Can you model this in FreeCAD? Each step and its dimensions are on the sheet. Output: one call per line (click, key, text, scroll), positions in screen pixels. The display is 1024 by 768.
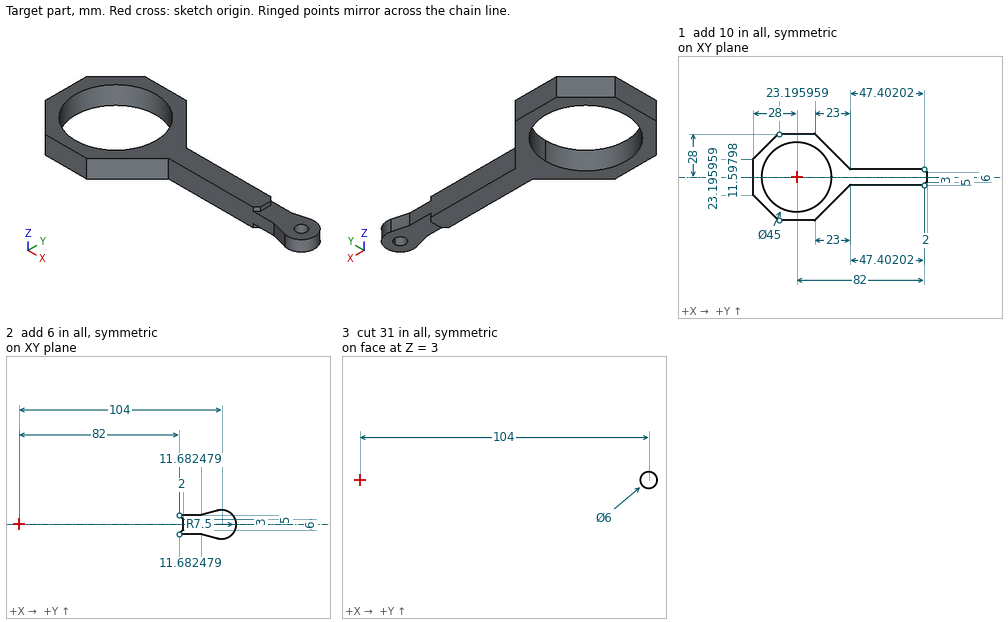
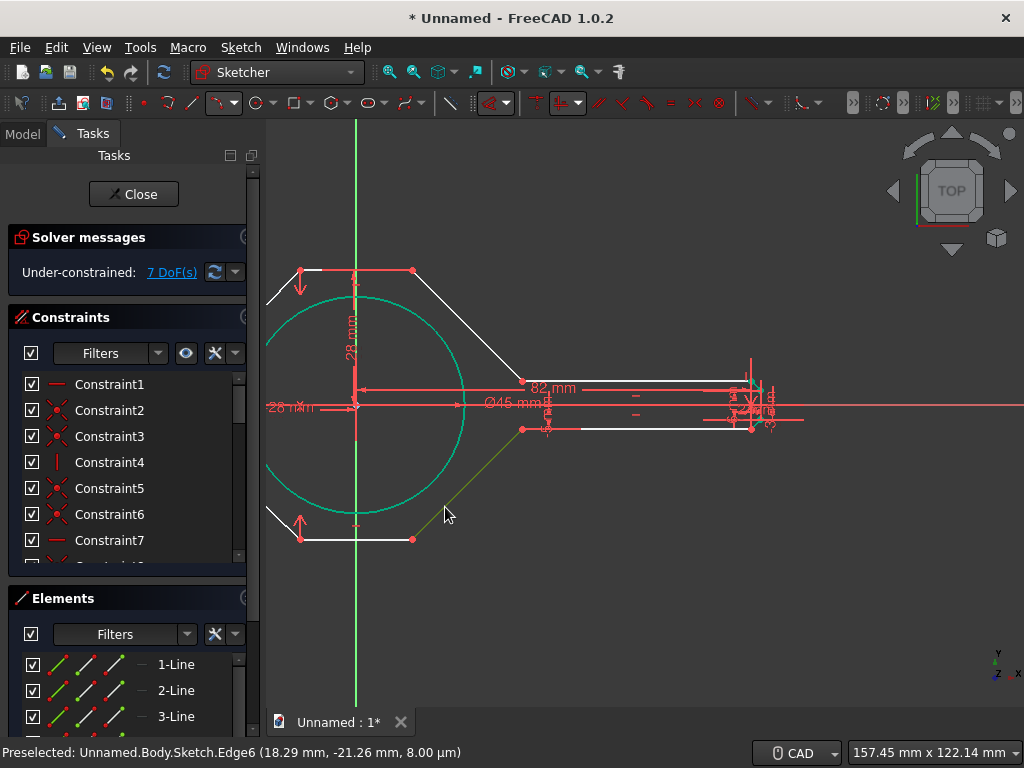
click(508, 104)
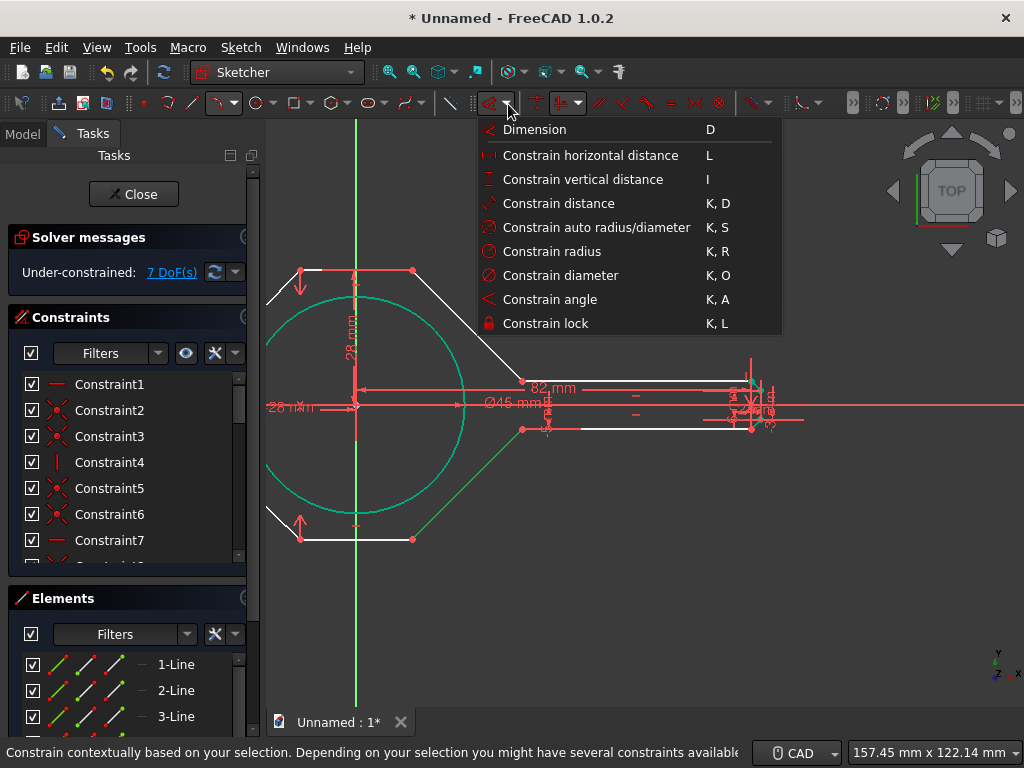
click(630, 155)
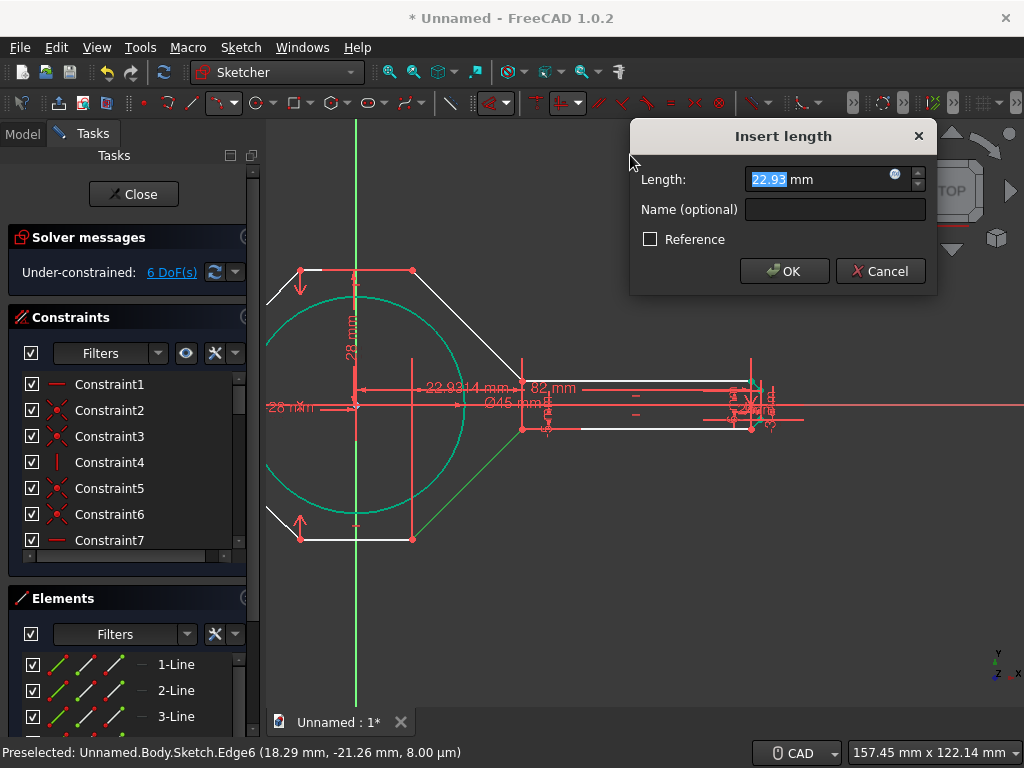
text(23)
key(Return)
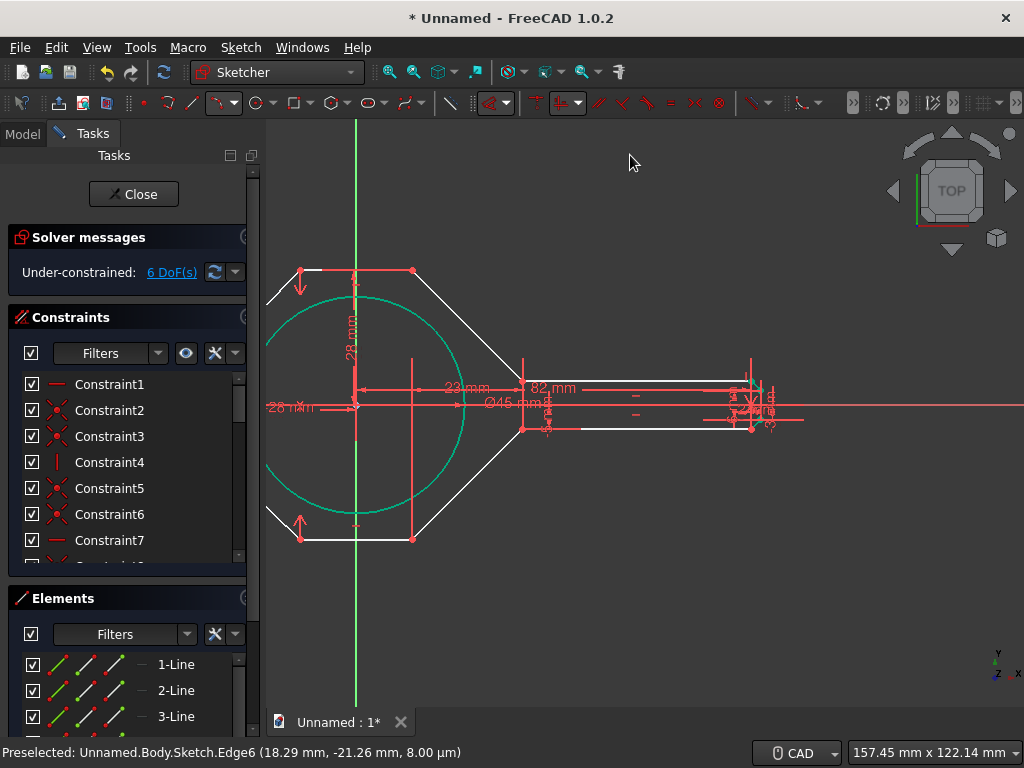
click(489, 348)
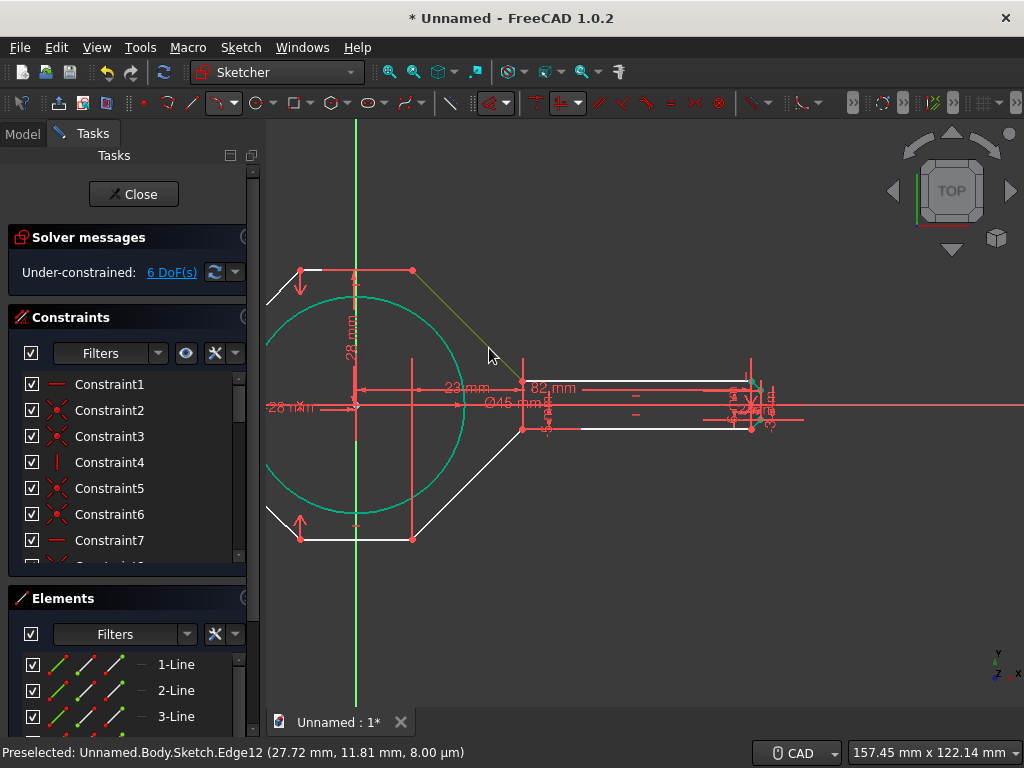
key(l)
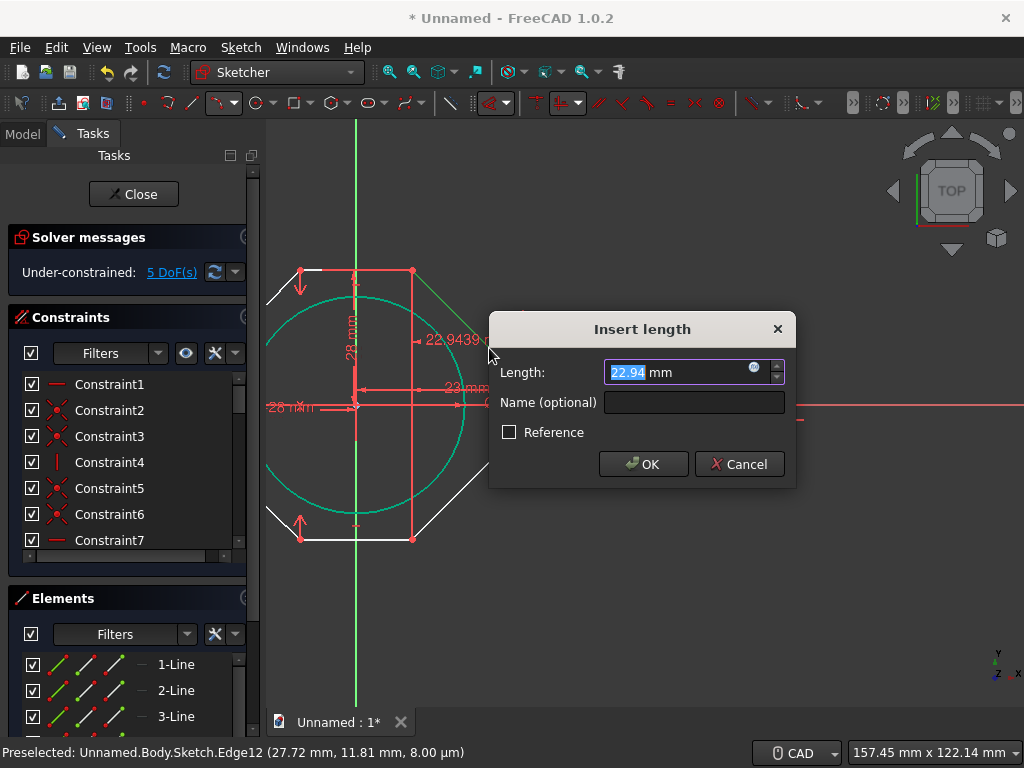
text(23)
key(Return)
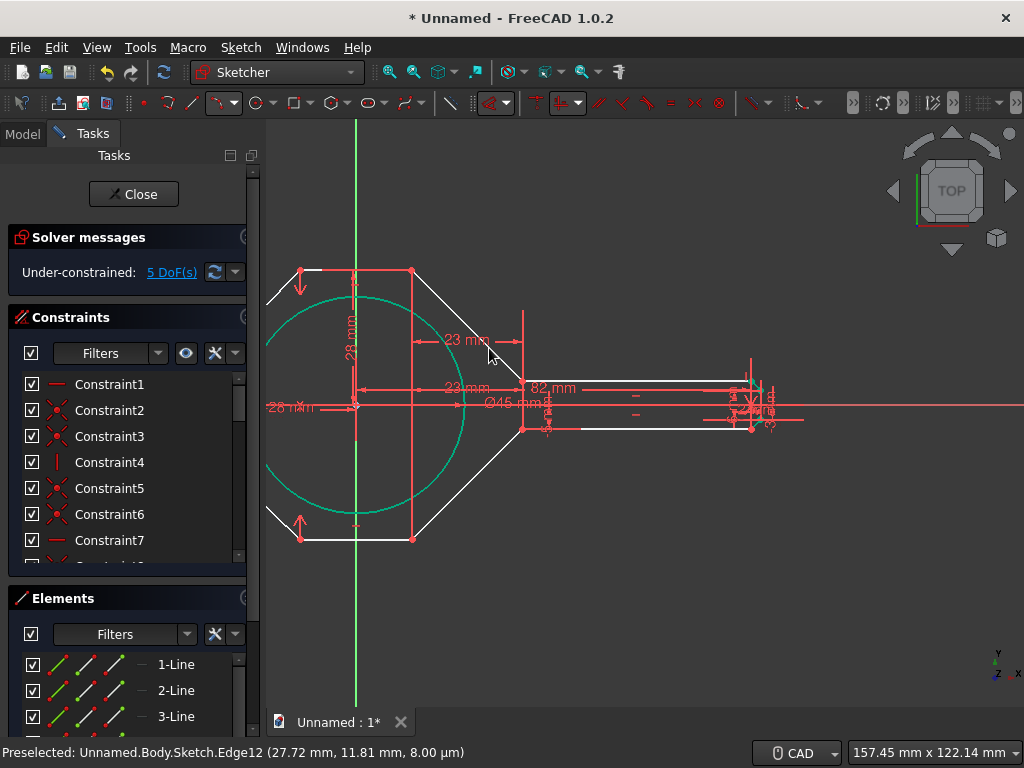
click(591, 429)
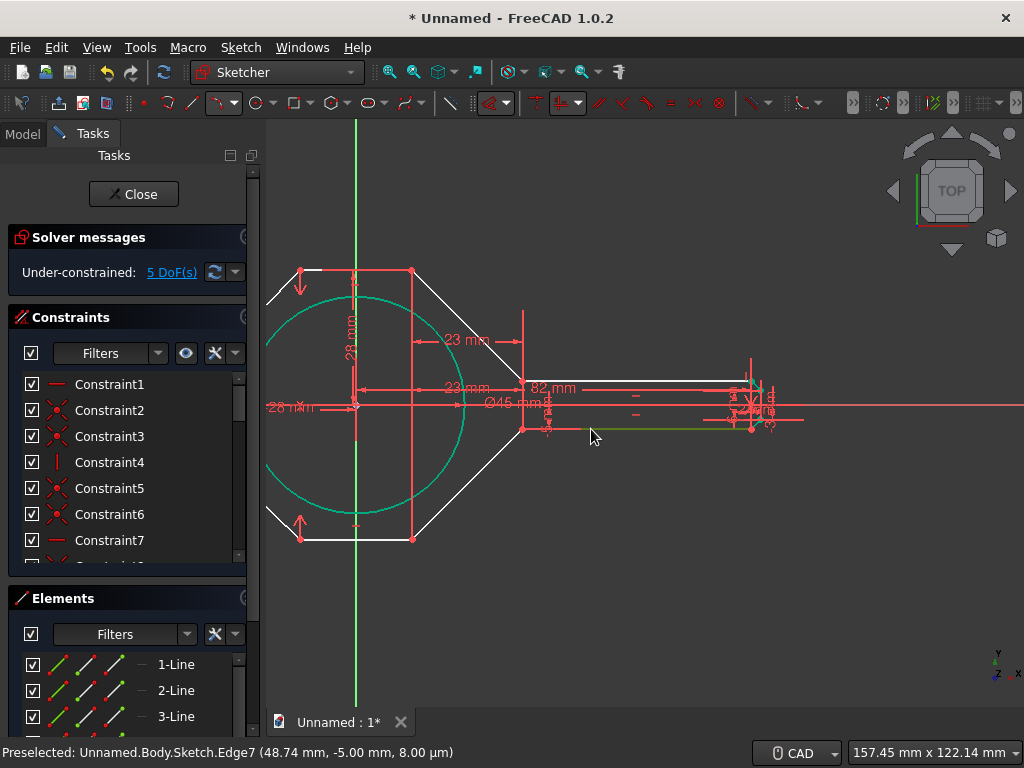
click(508, 104)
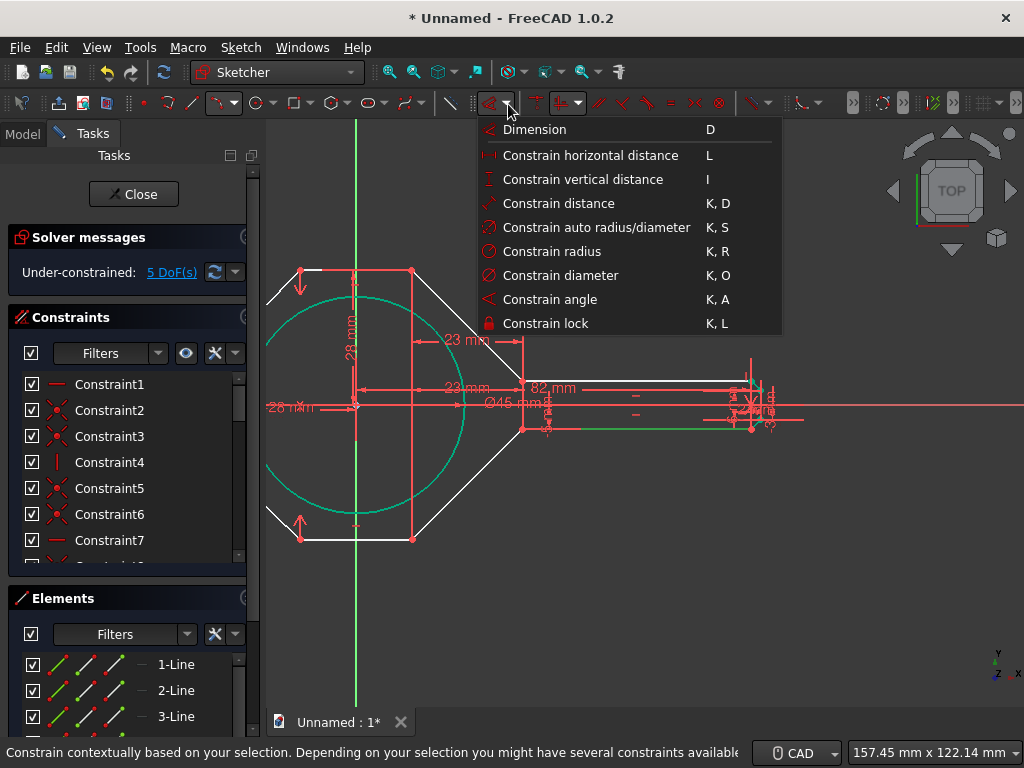
click(630, 155)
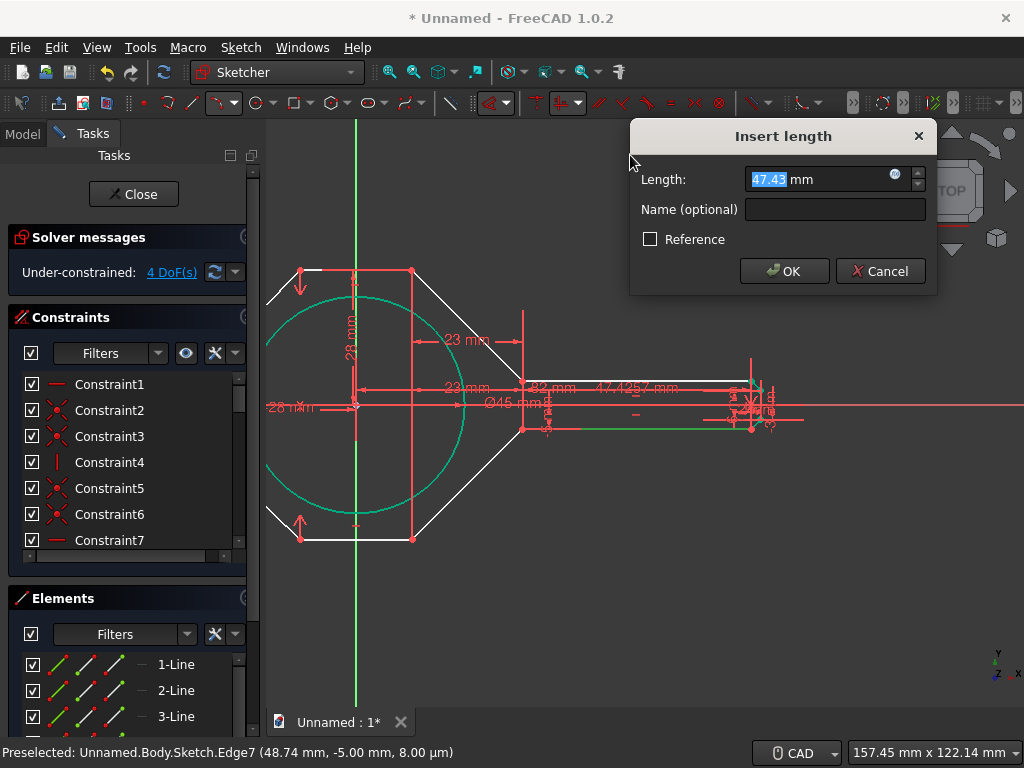
text(47.40202)
key(Return)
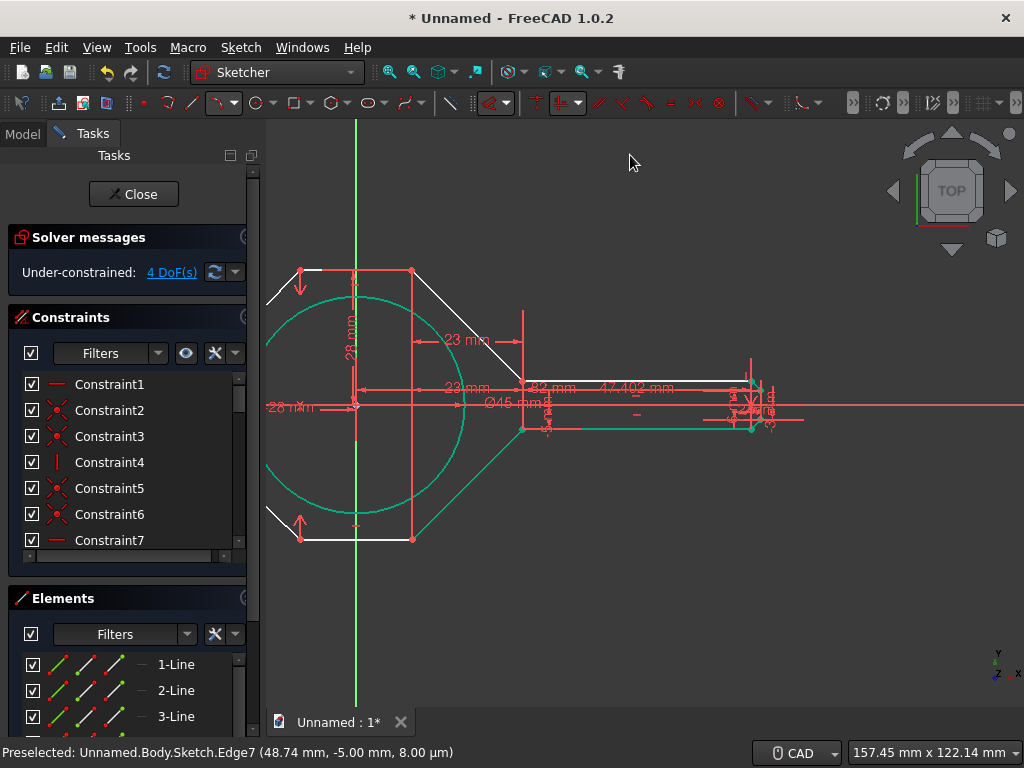
click(683, 381)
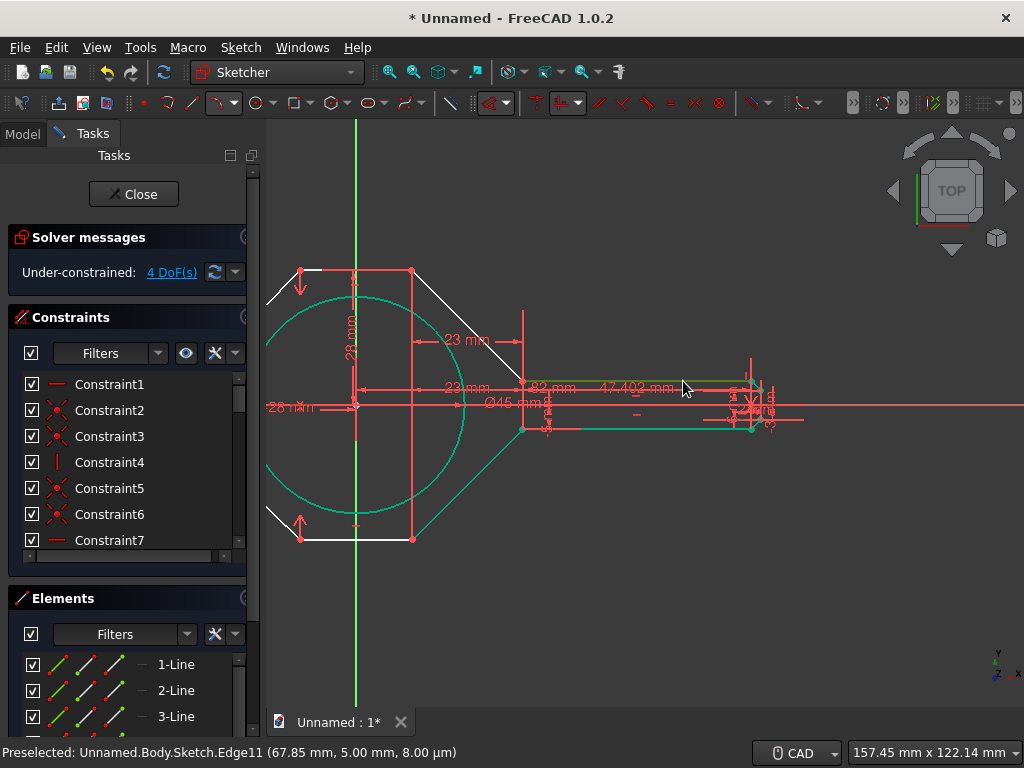
key(l)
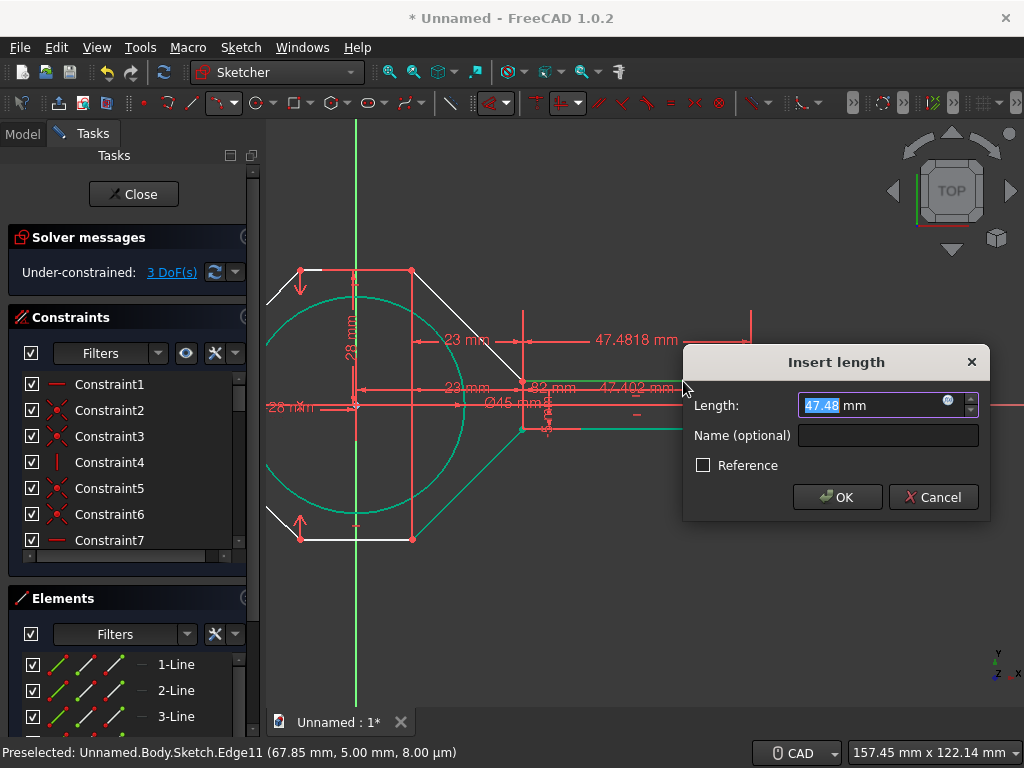
text(47.40202)
key(Return)